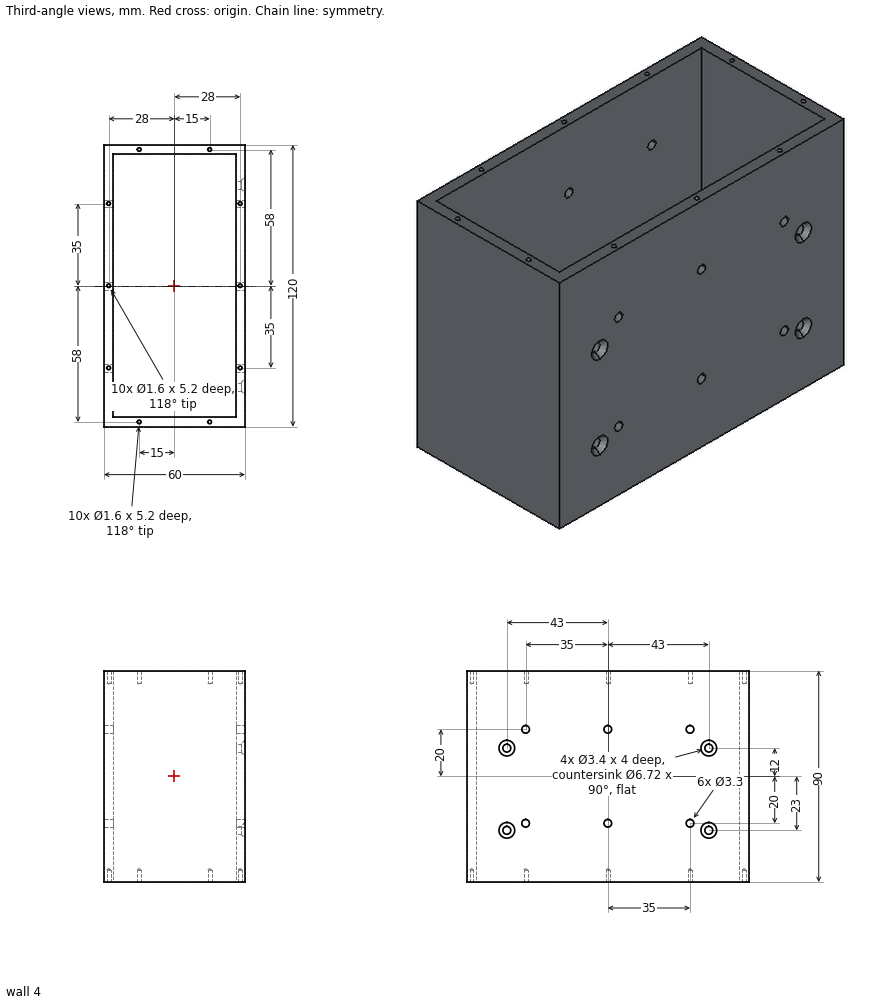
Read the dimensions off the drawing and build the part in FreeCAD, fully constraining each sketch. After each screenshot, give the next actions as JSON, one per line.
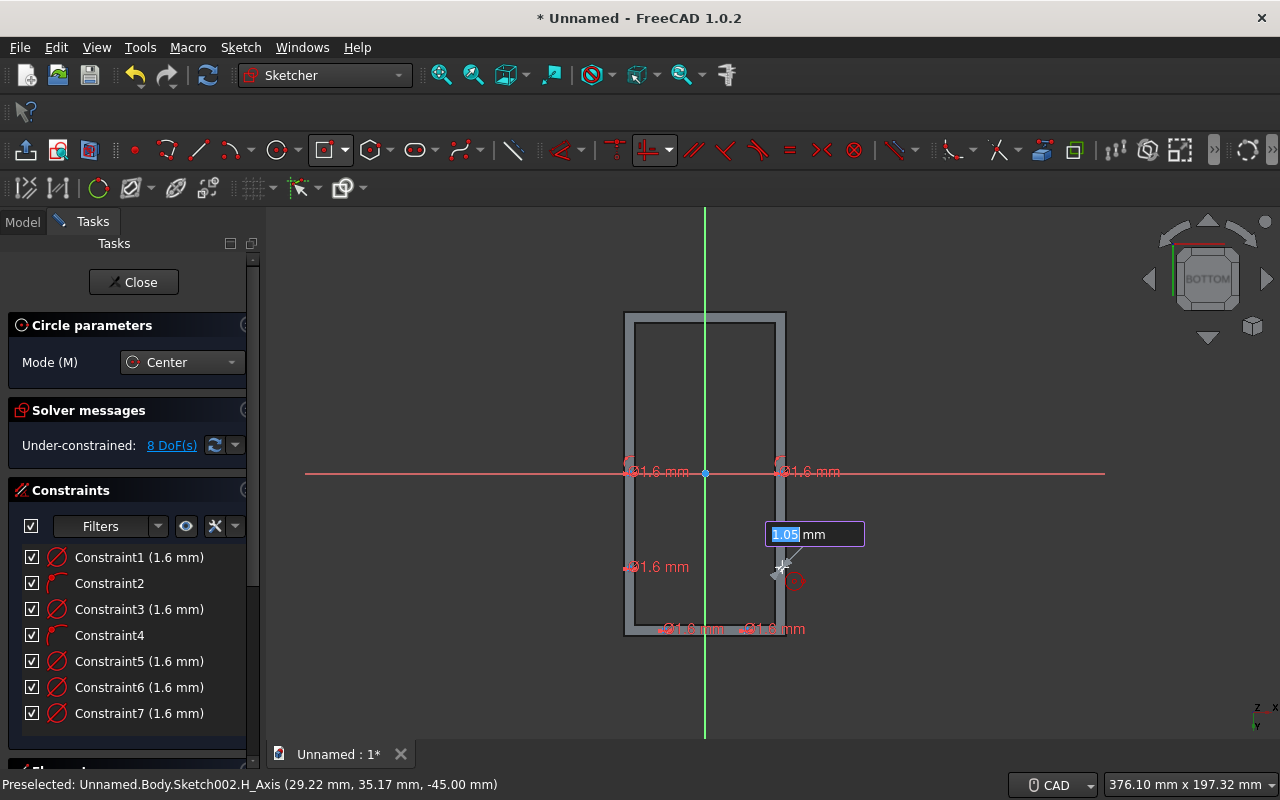
{"action": "type", "text": "1.6"}
{"action": "key", "text": "Return"}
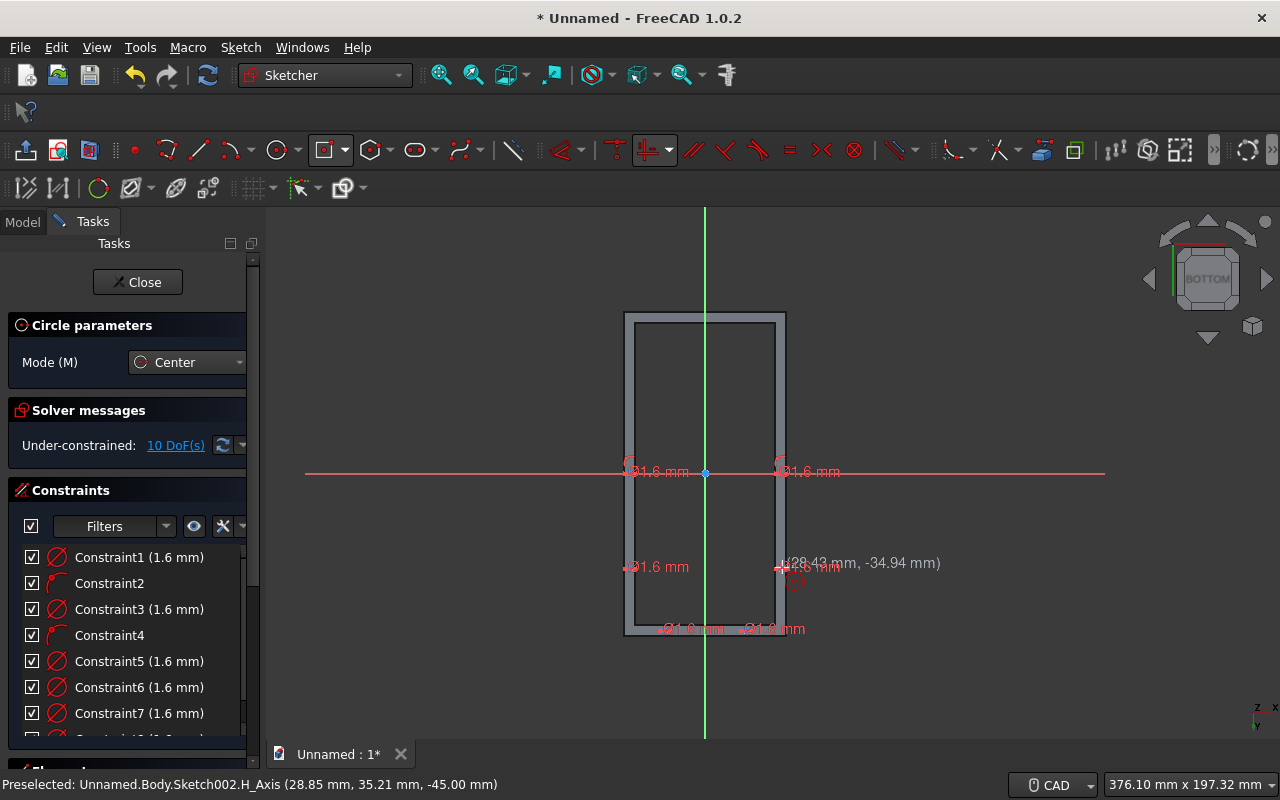
{"action": "scroll", "coordinate": [781, 379], "scroll_direction": "up", "scroll_amount": 12}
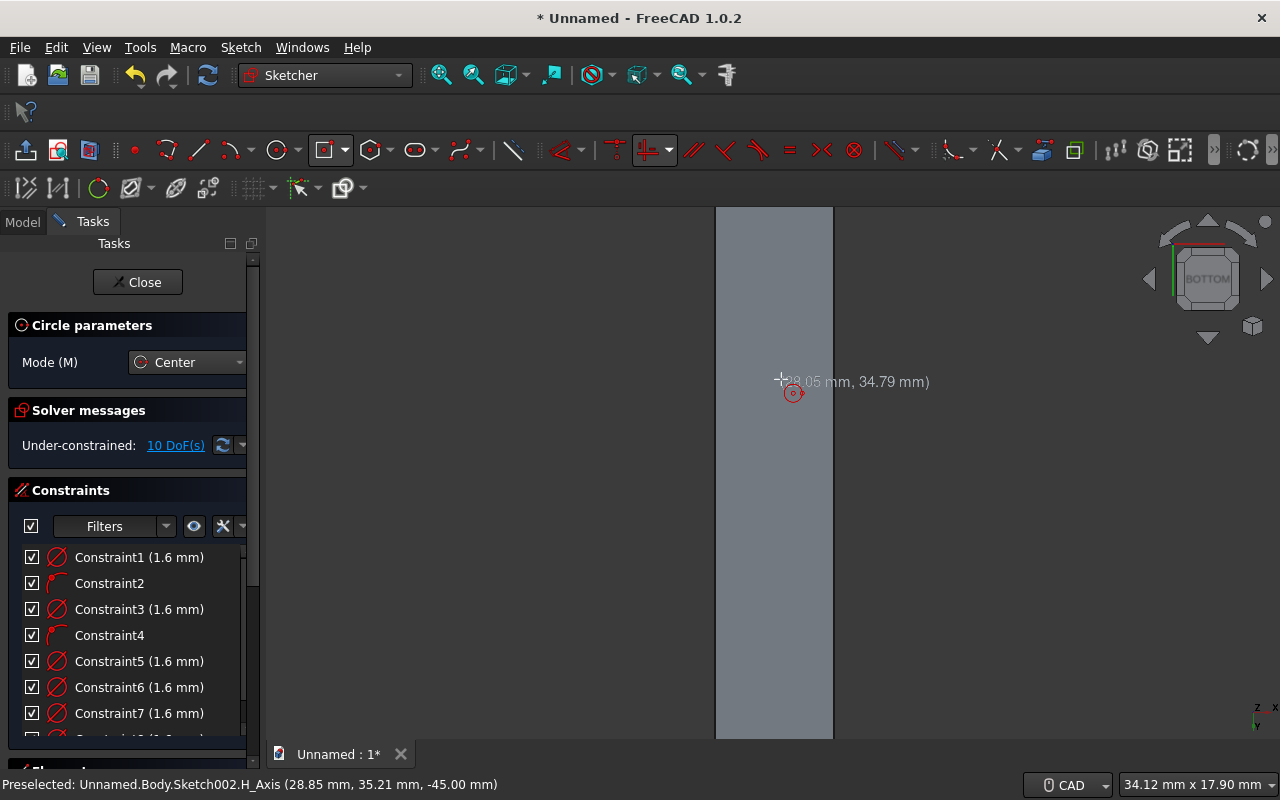
{"action": "scroll", "coordinate": [781, 378], "scroll_direction": "down", "scroll_amount": 12}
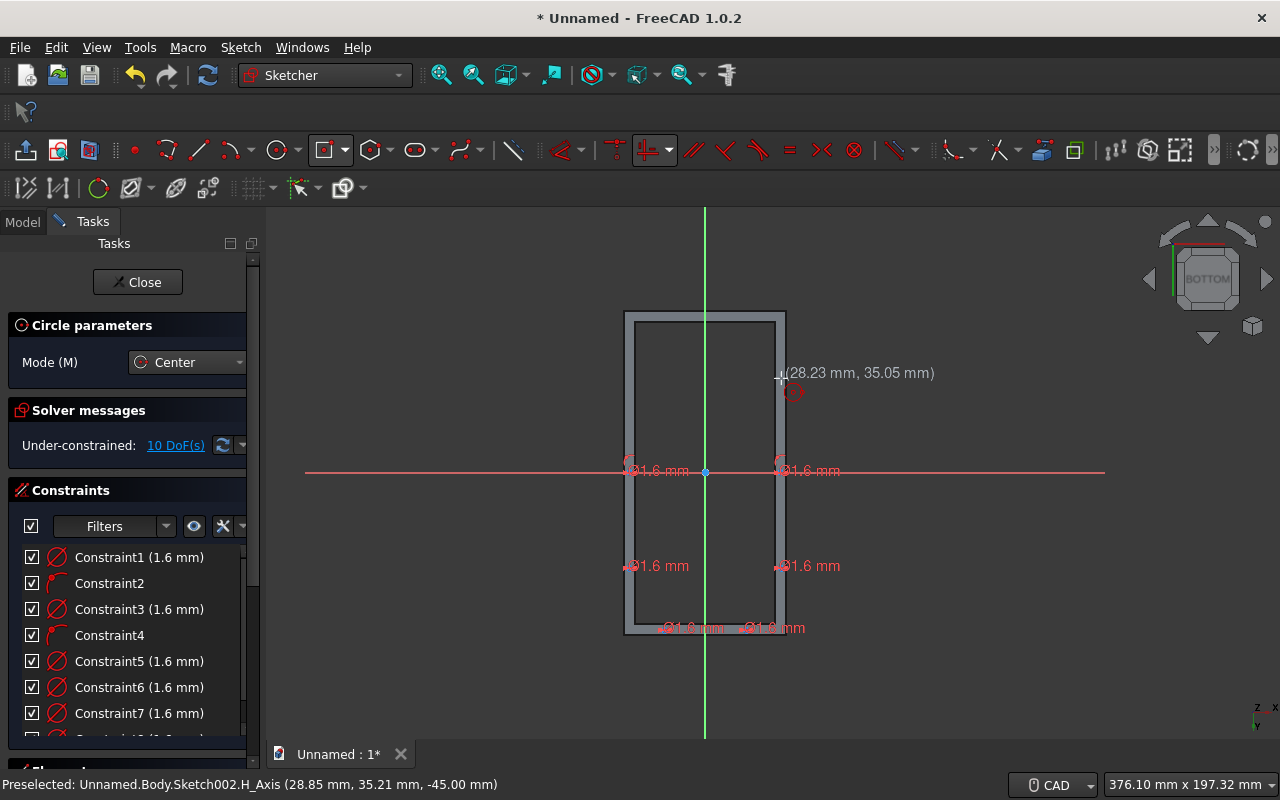
{"action": "left_click", "coordinate": [781, 379]}
{"action": "mouse_move", "coordinate": [782, 377]}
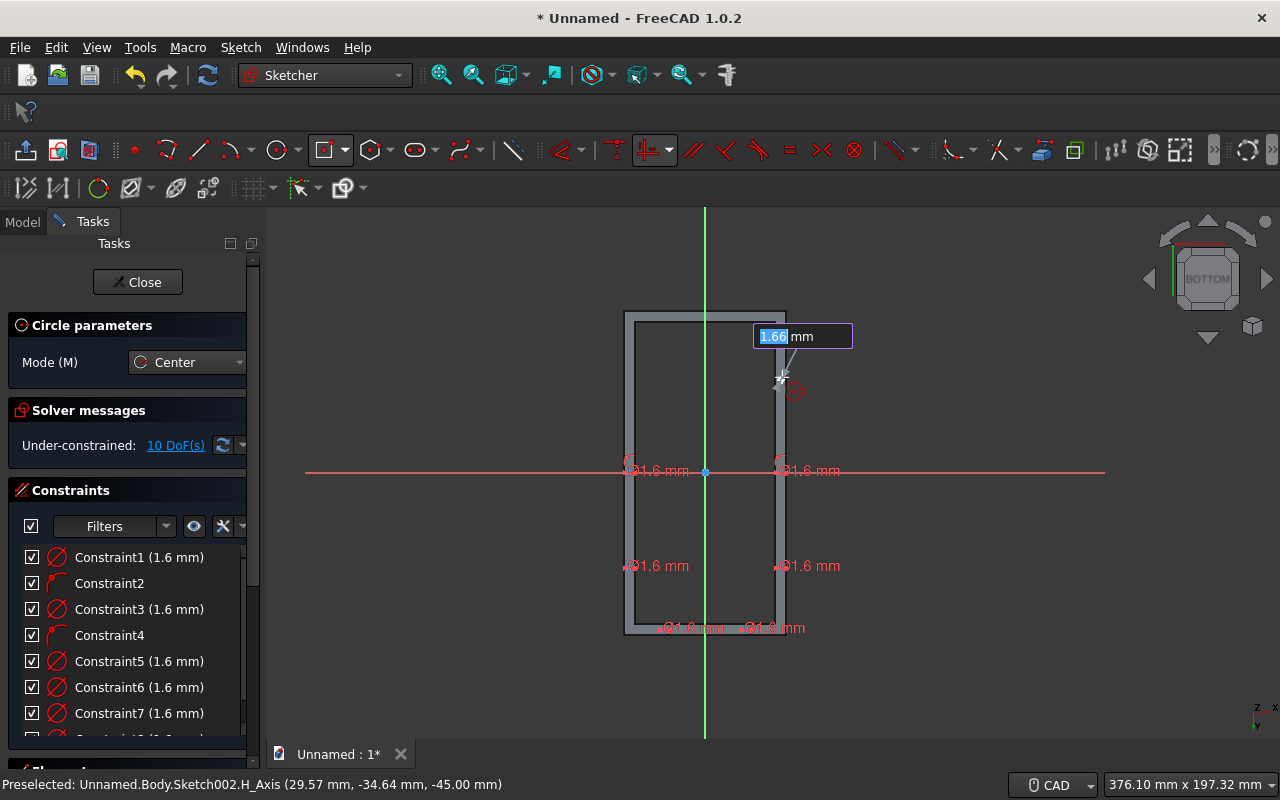
{"action": "type", "text": "1.6"}
{"action": "key", "text": "Return"}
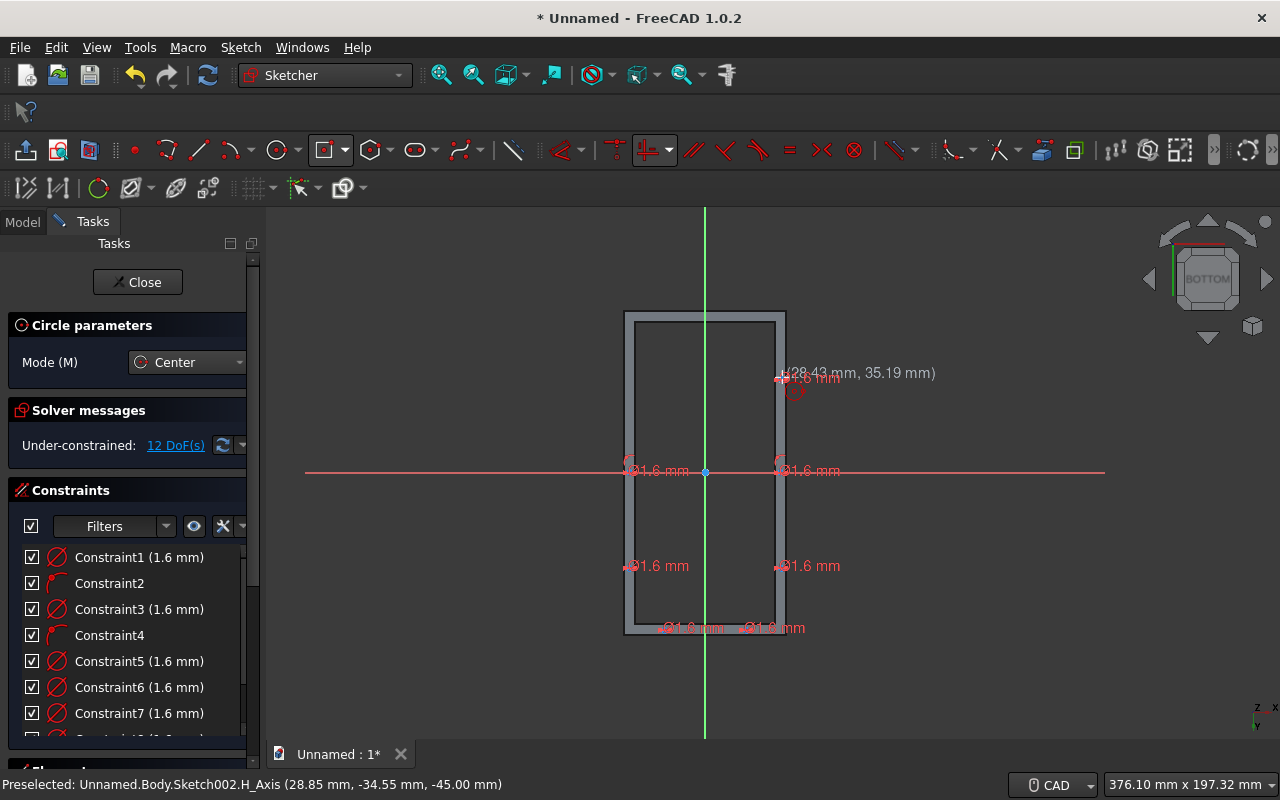
{"action": "scroll", "coordinate": [630, 379], "scroll_direction": "up", "scroll_amount": 12}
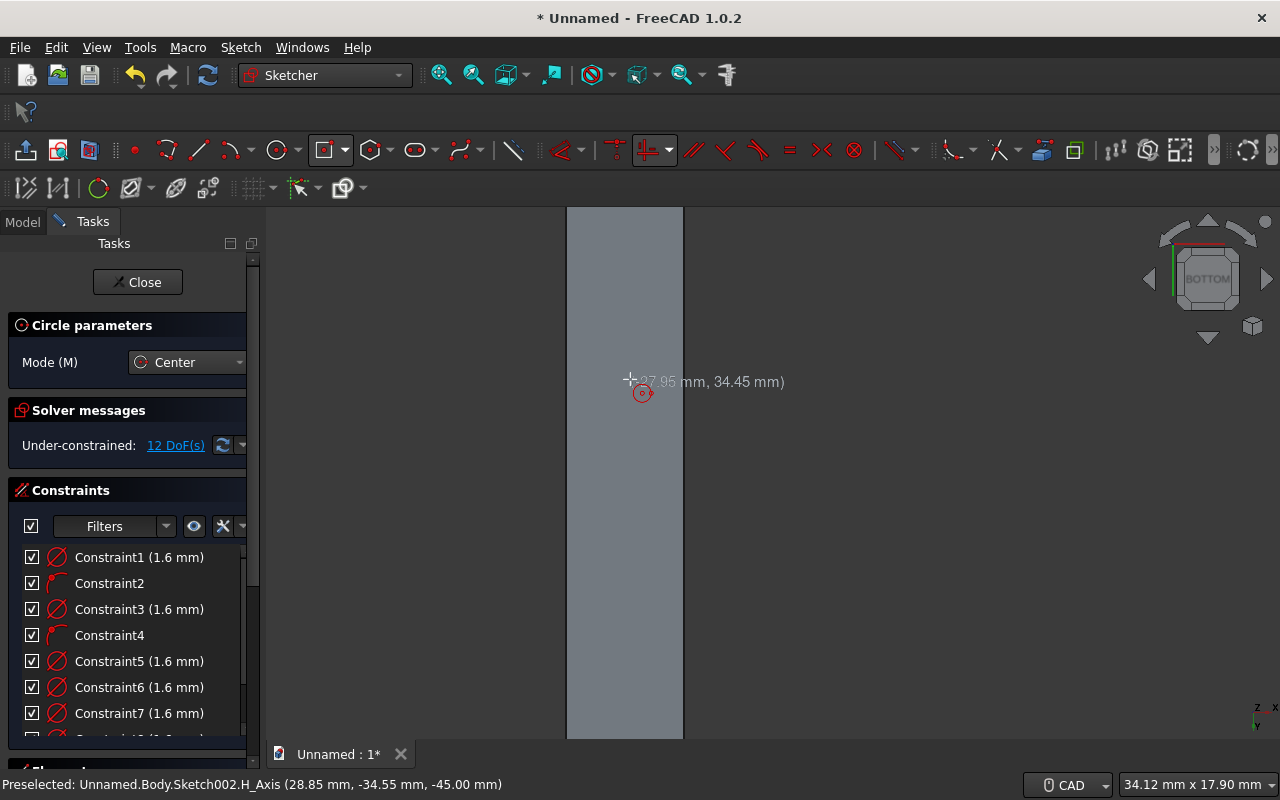
{"action": "scroll", "coordinate": [629, 379], "scroll_direction": "down", "scroll_amount": 12}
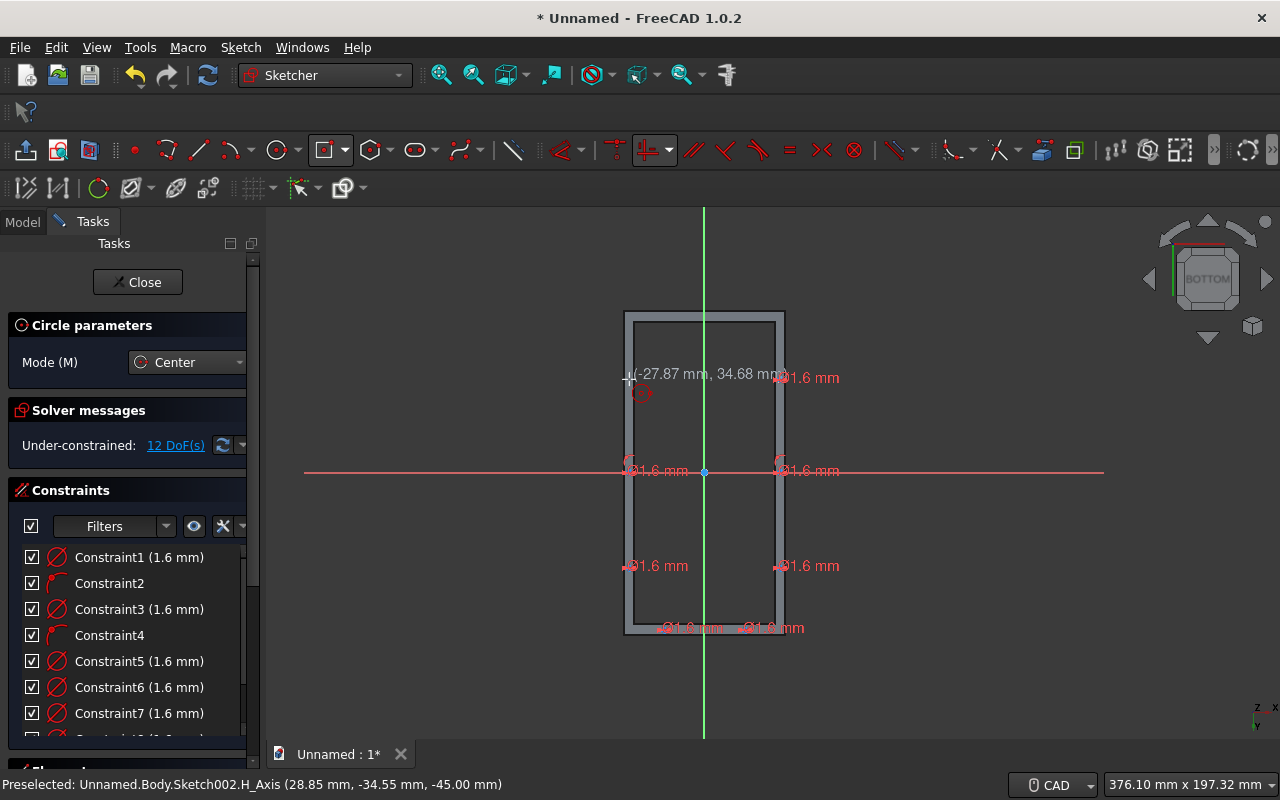
{"action": "left_click", "coordinate": [629, 379]}
{"action": "mouse_move", "coordinate": [630, 377]}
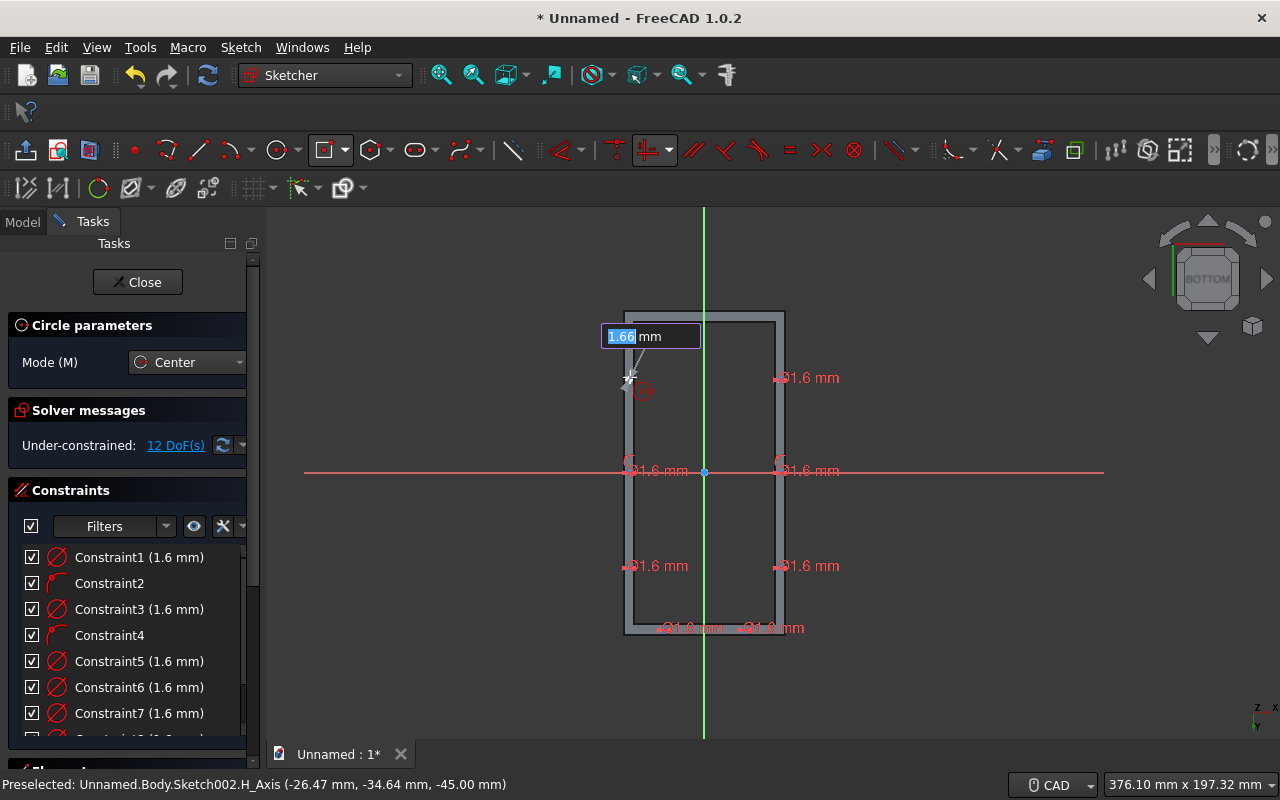
{"action": "type", "text": "1.6"}
{"action": "key", "text": "Return"}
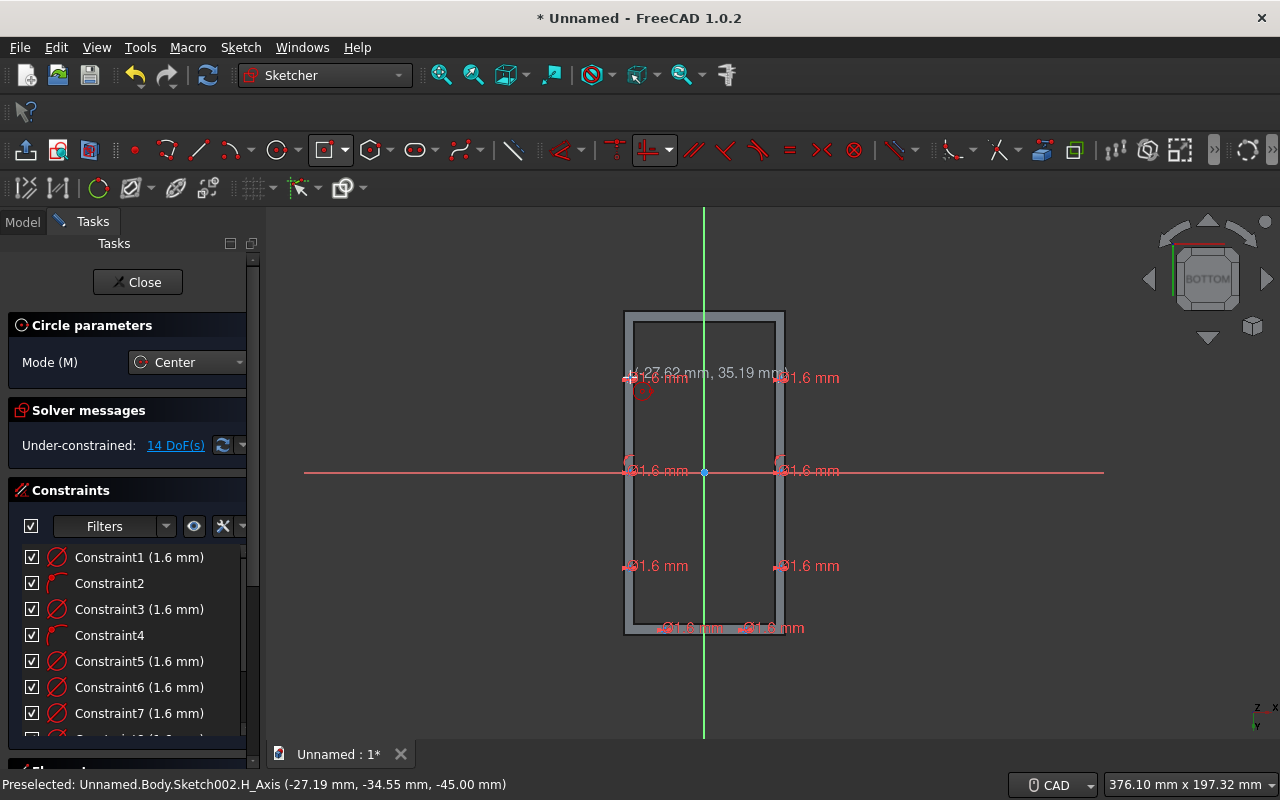
{"action": "scroll", "coordinate": [745, 317], "scroll_direction": "up", "scroll_amount": 12}